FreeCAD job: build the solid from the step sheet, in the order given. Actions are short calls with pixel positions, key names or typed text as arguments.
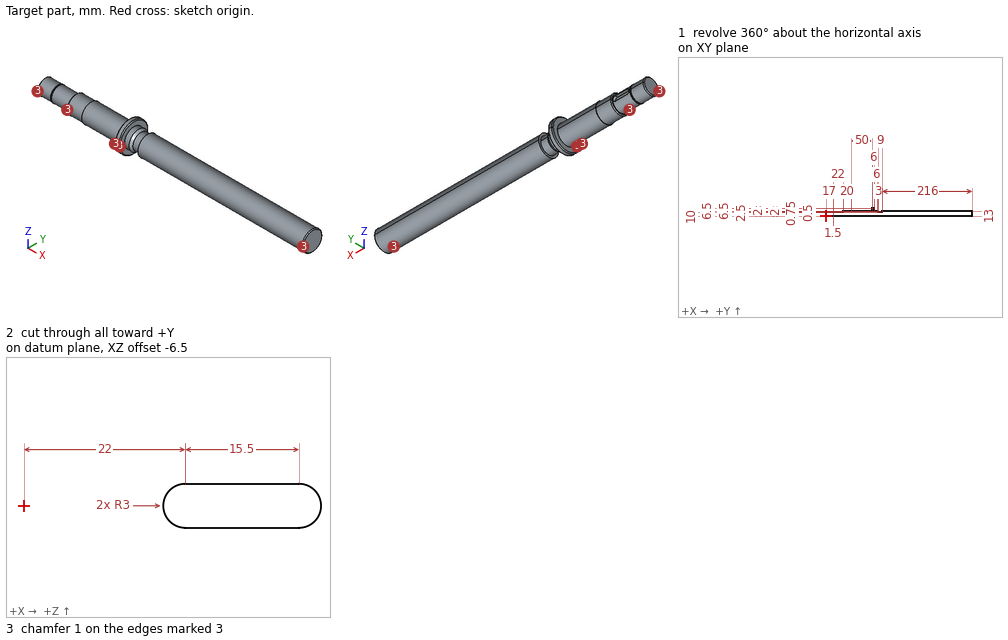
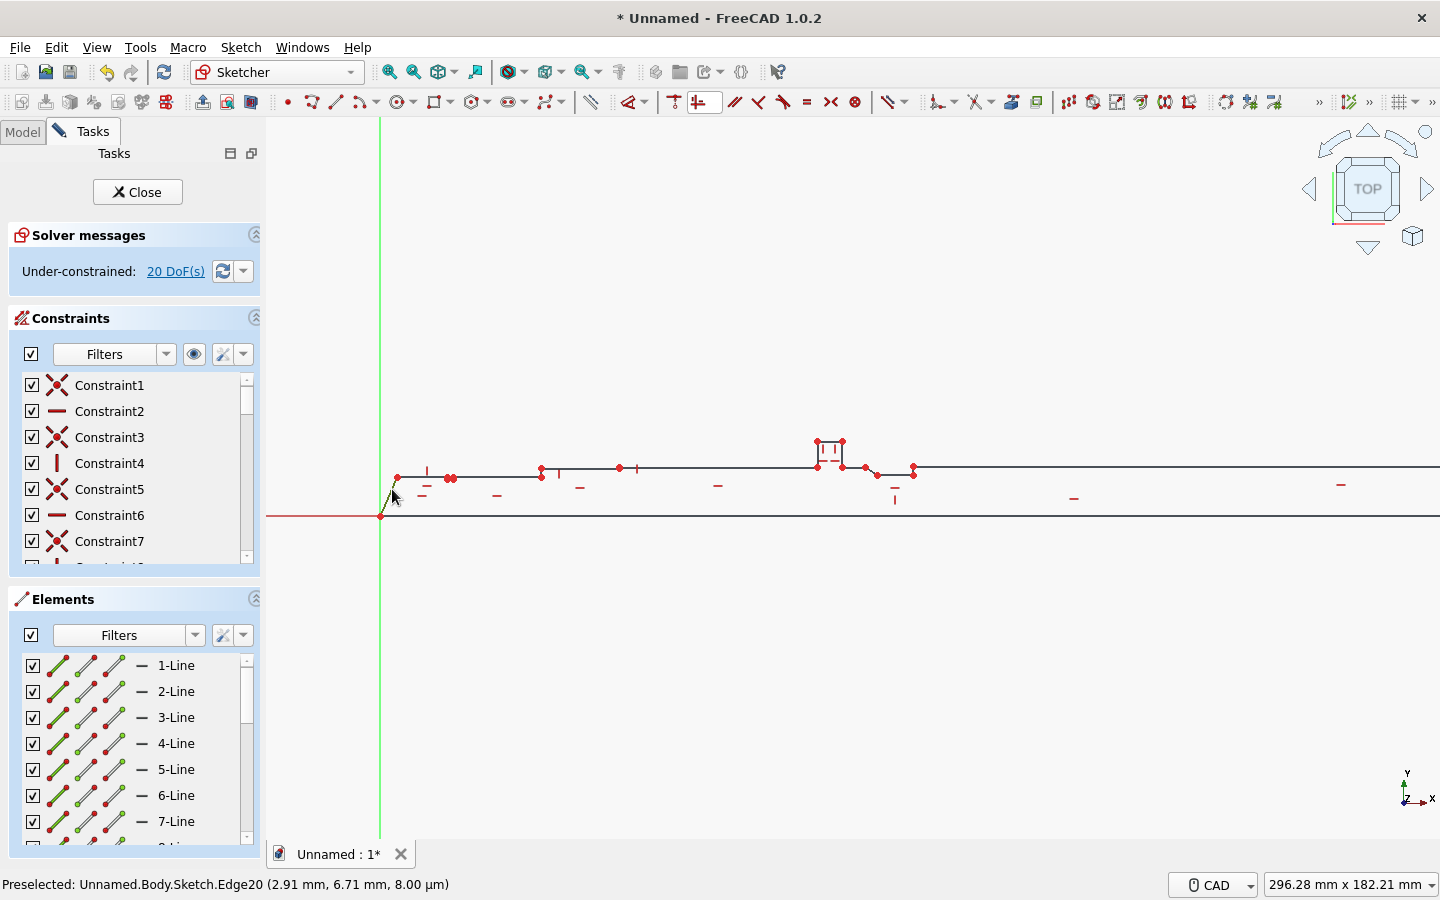
key(v)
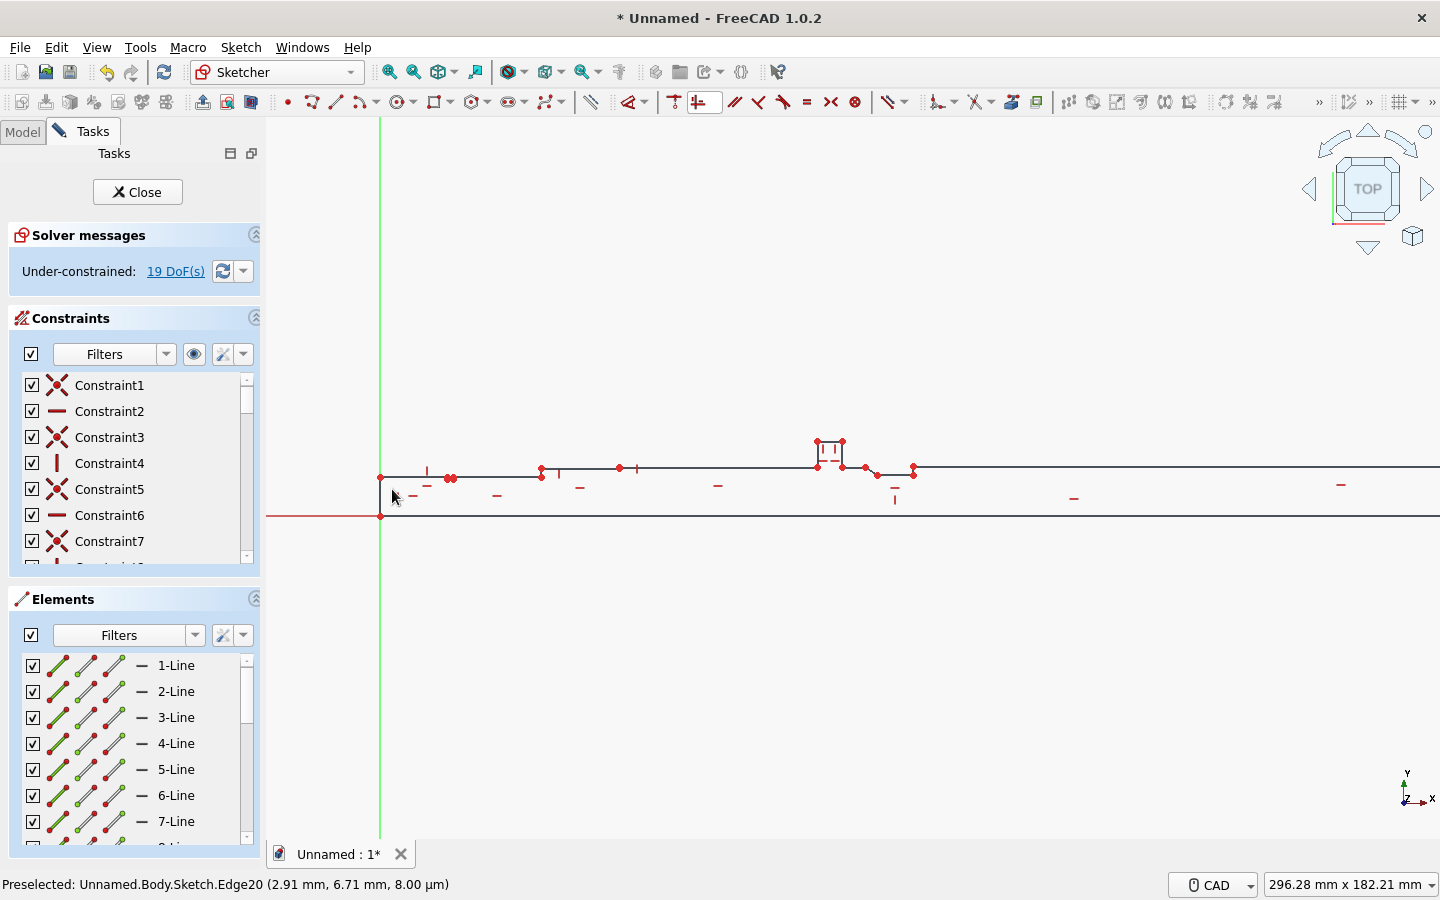
click(628, 102)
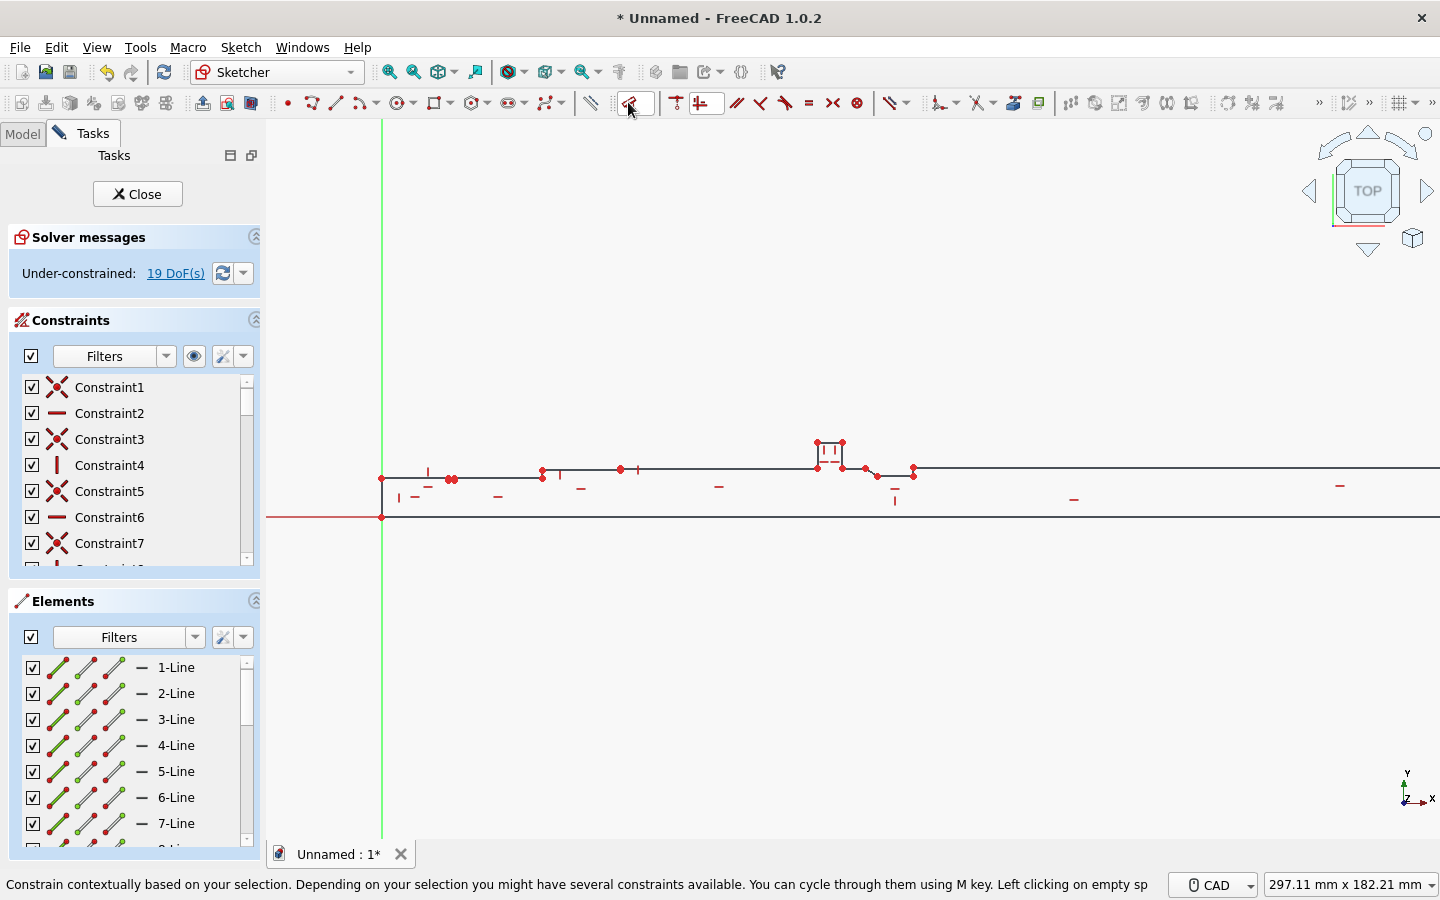
scroll(903, 476, up, 2)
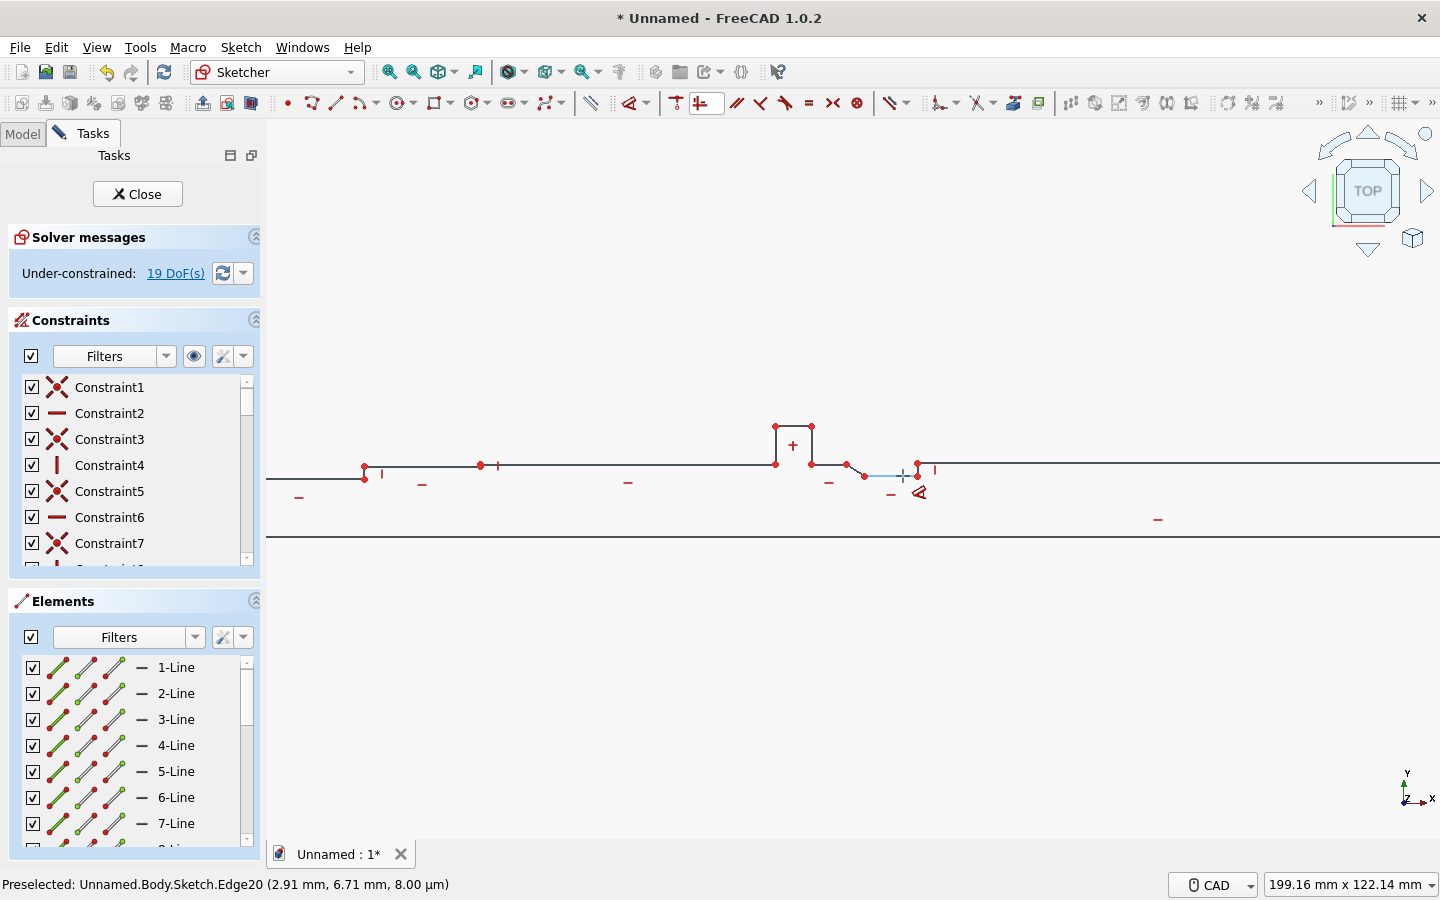
click(902, 476)
click(891, 442)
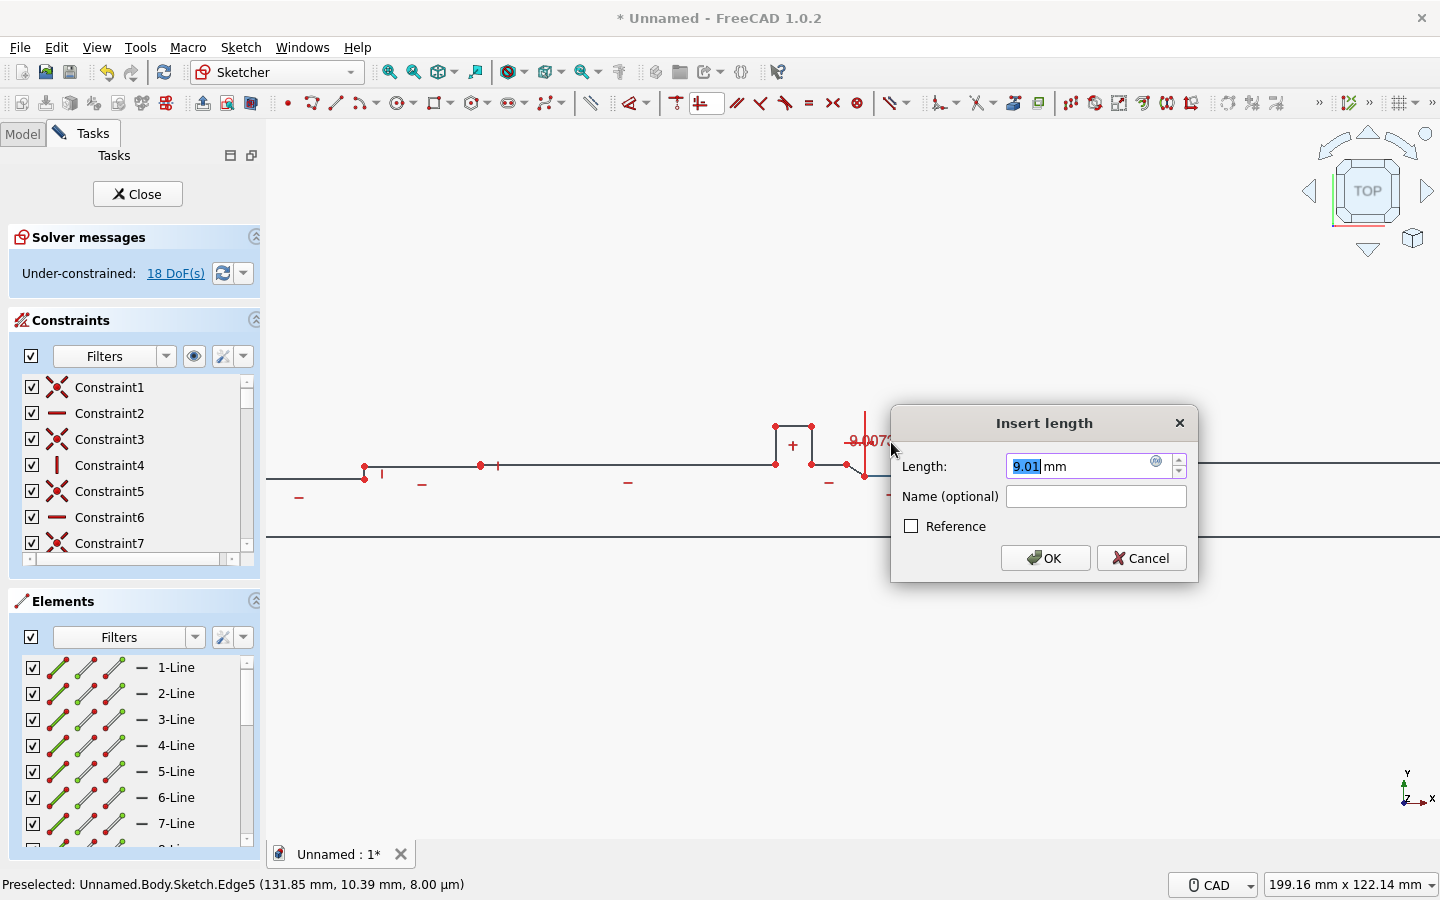
text(9)
key(Return)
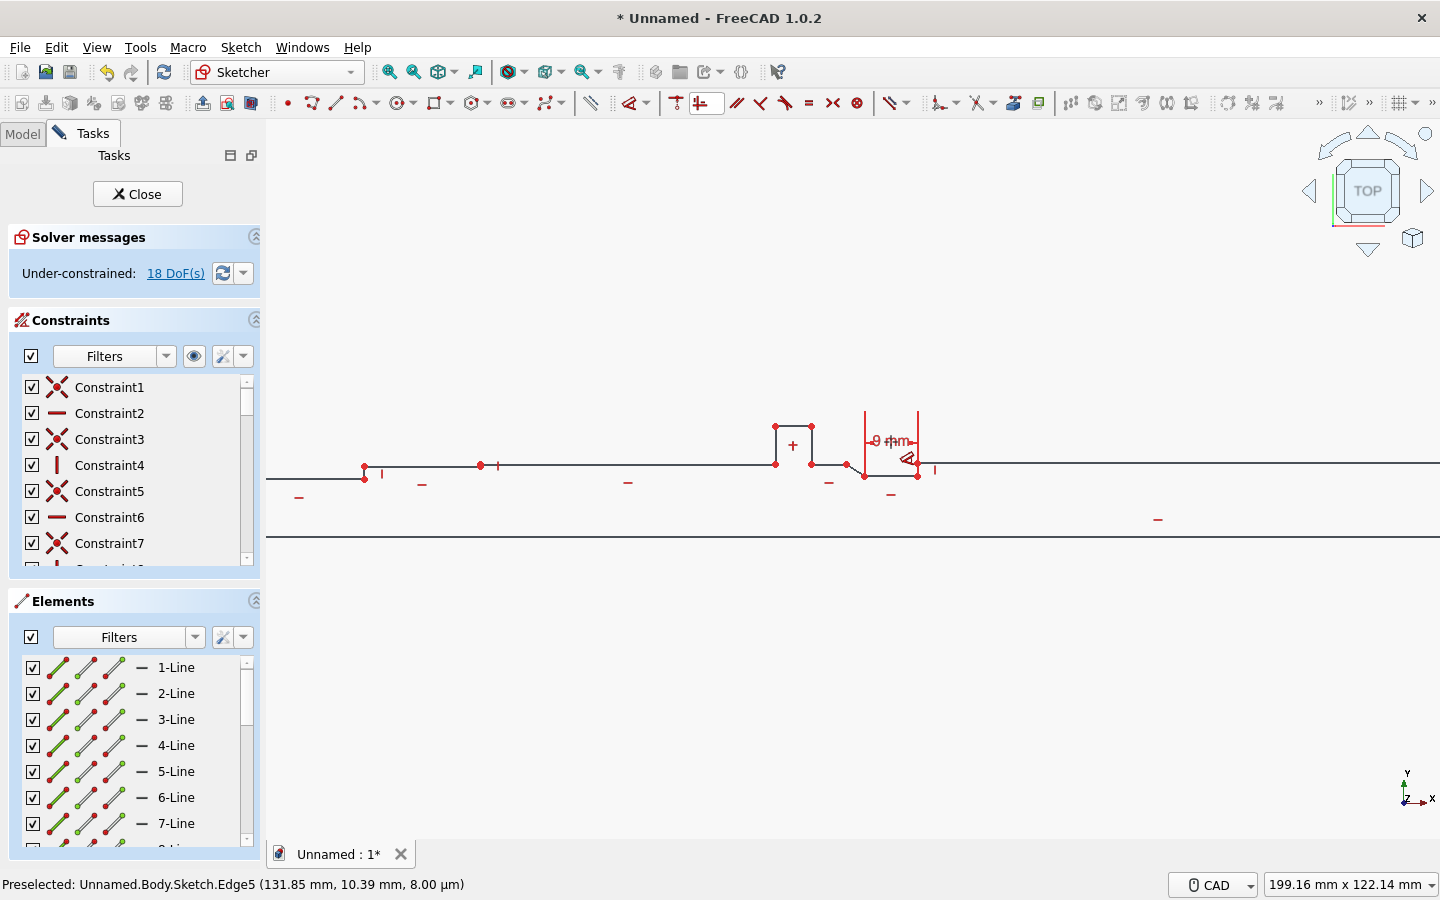
scroll(836, 465, up, 2)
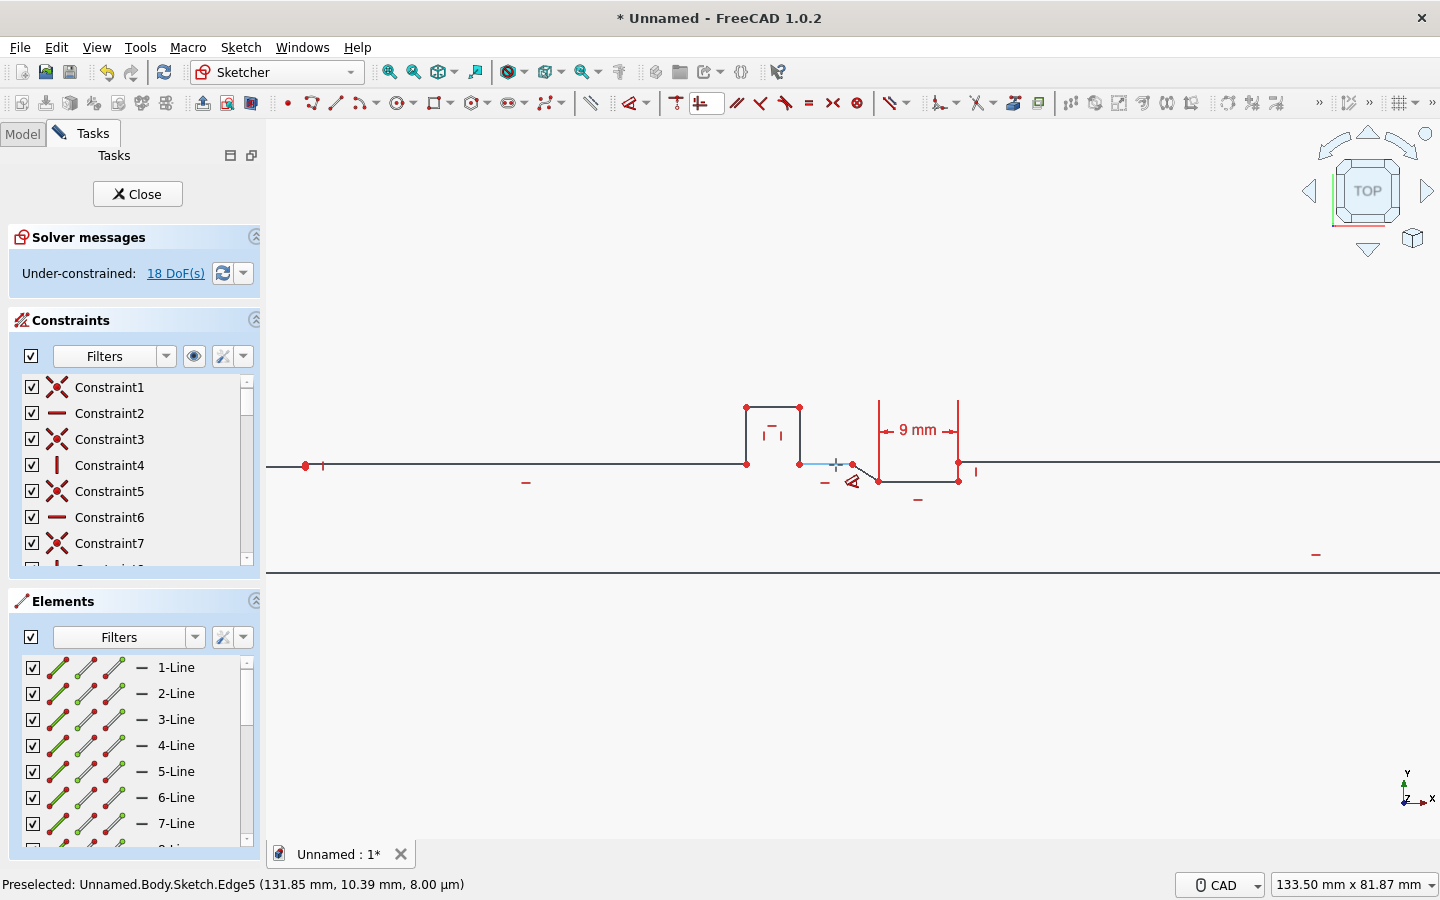
click(836, 464)
click(826, 430)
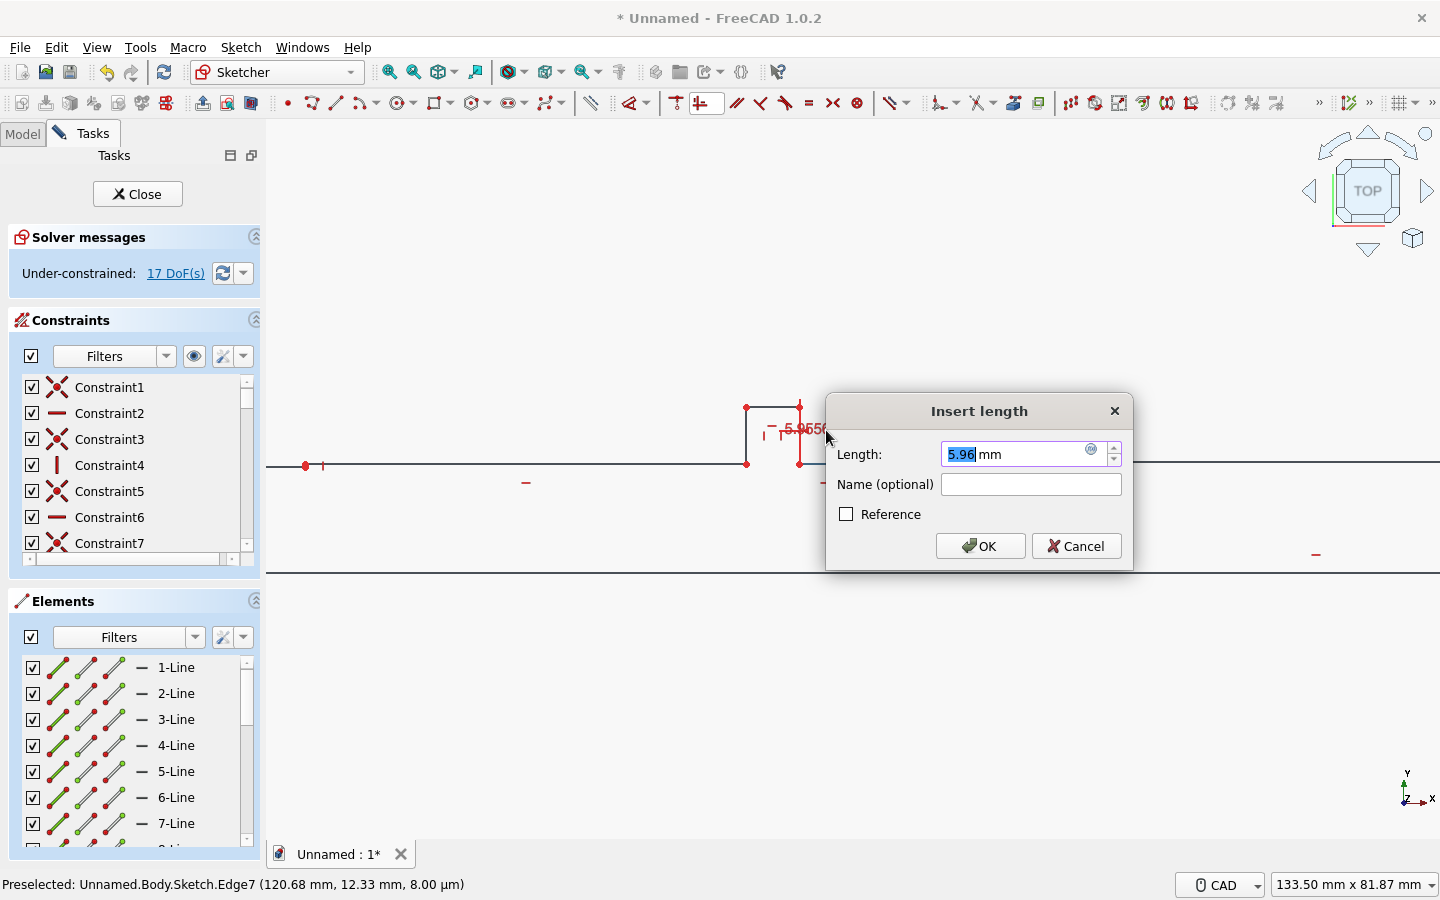
text(6)
key(Return)